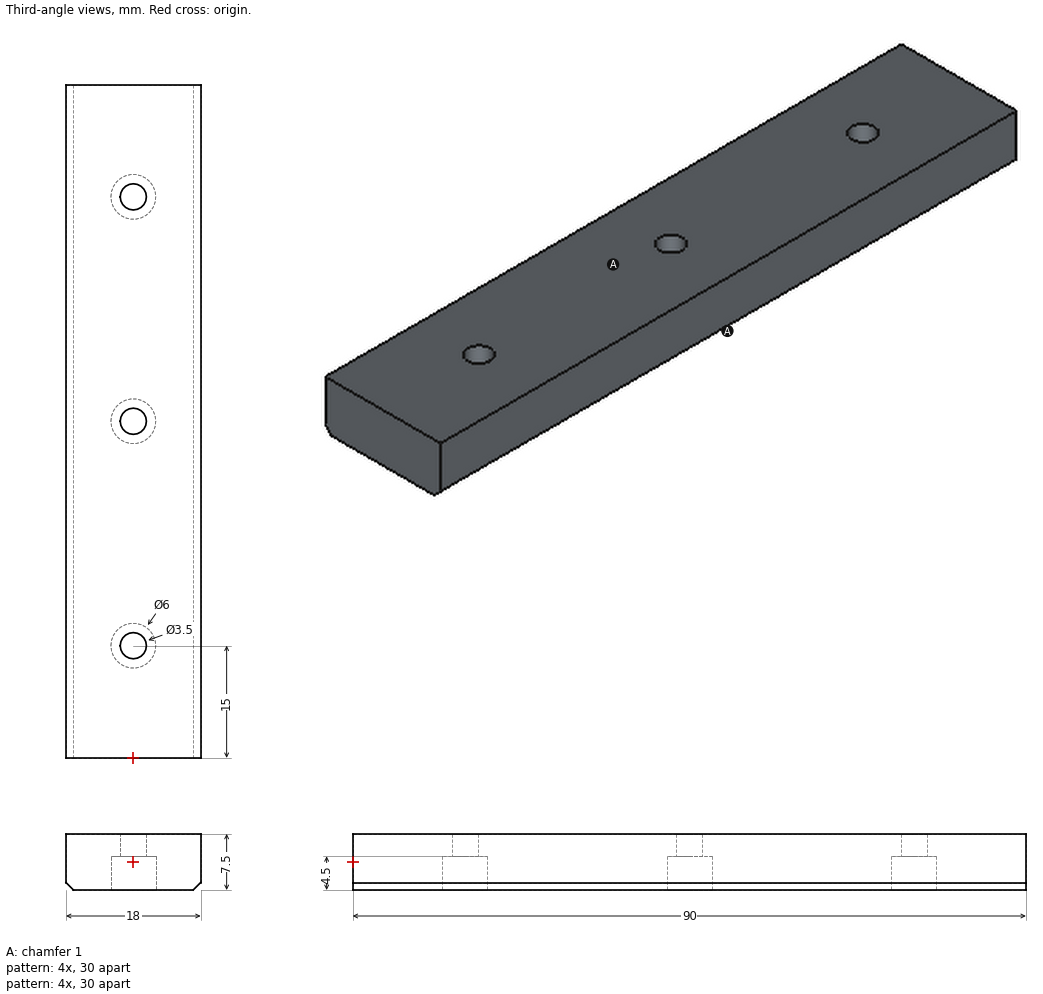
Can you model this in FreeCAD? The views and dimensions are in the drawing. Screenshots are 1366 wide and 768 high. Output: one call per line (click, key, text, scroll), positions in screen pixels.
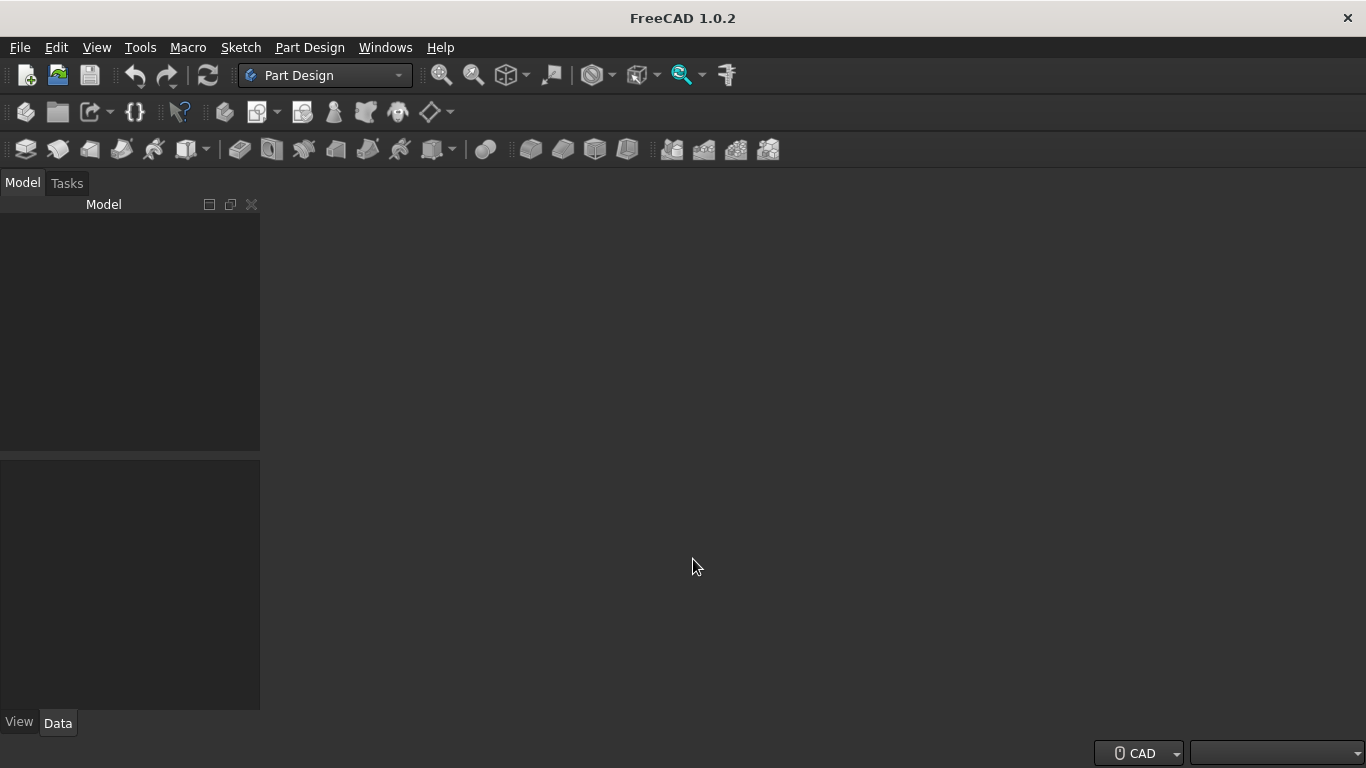
click(26, 76)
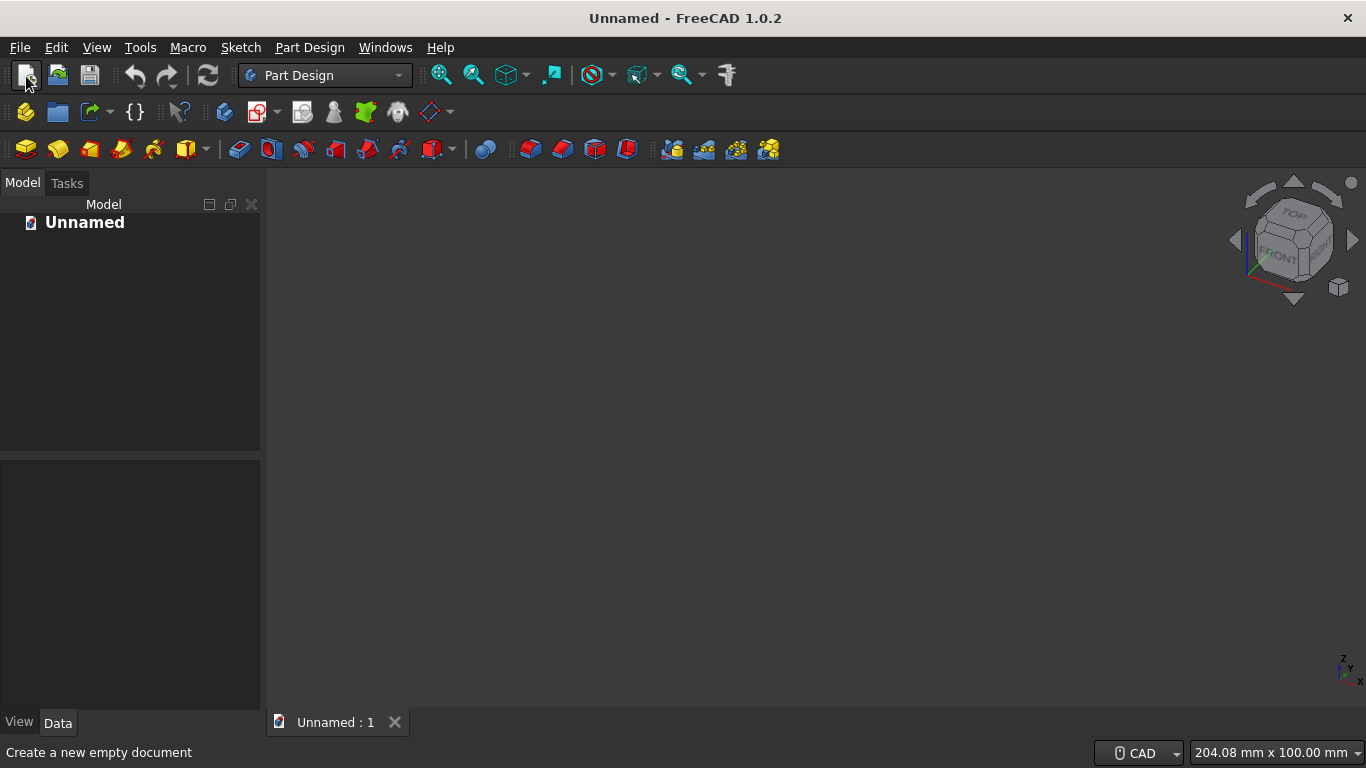
click(258, 112)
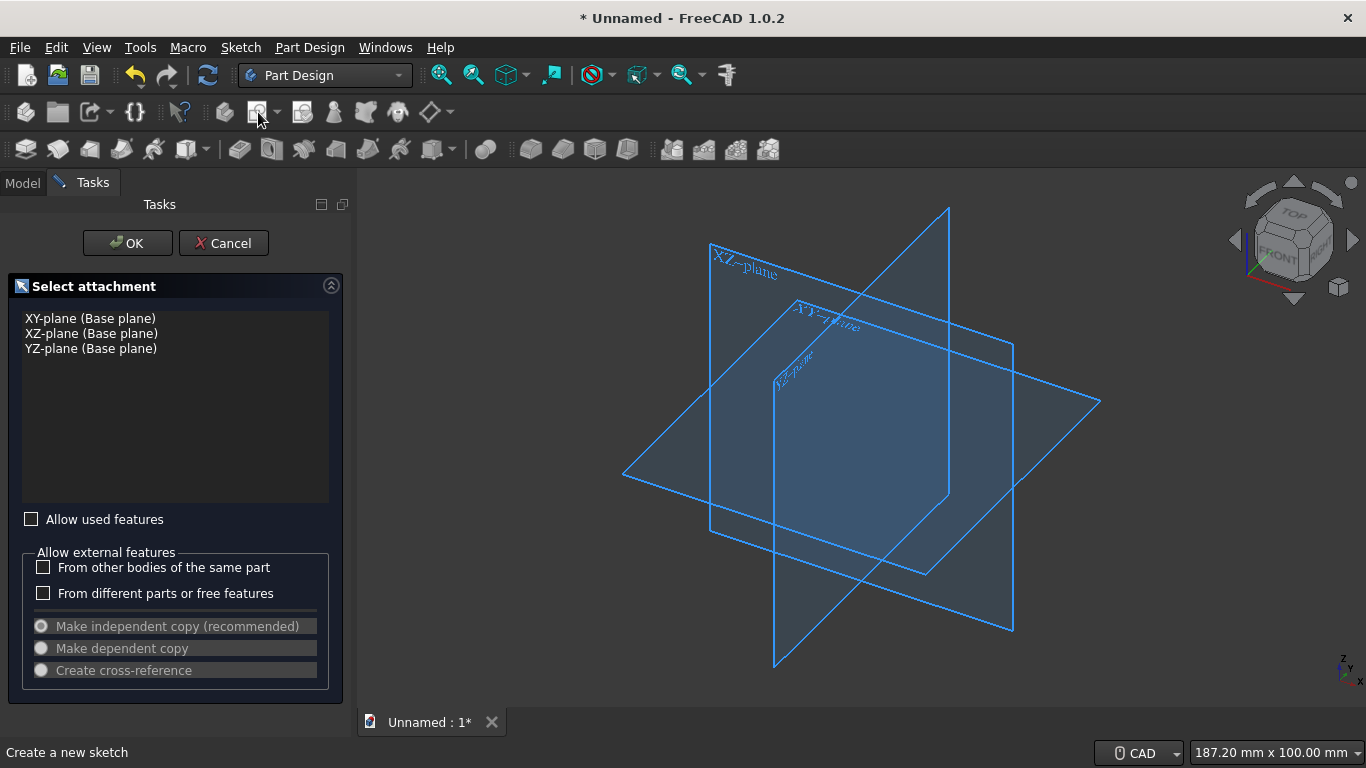
click(82, 334)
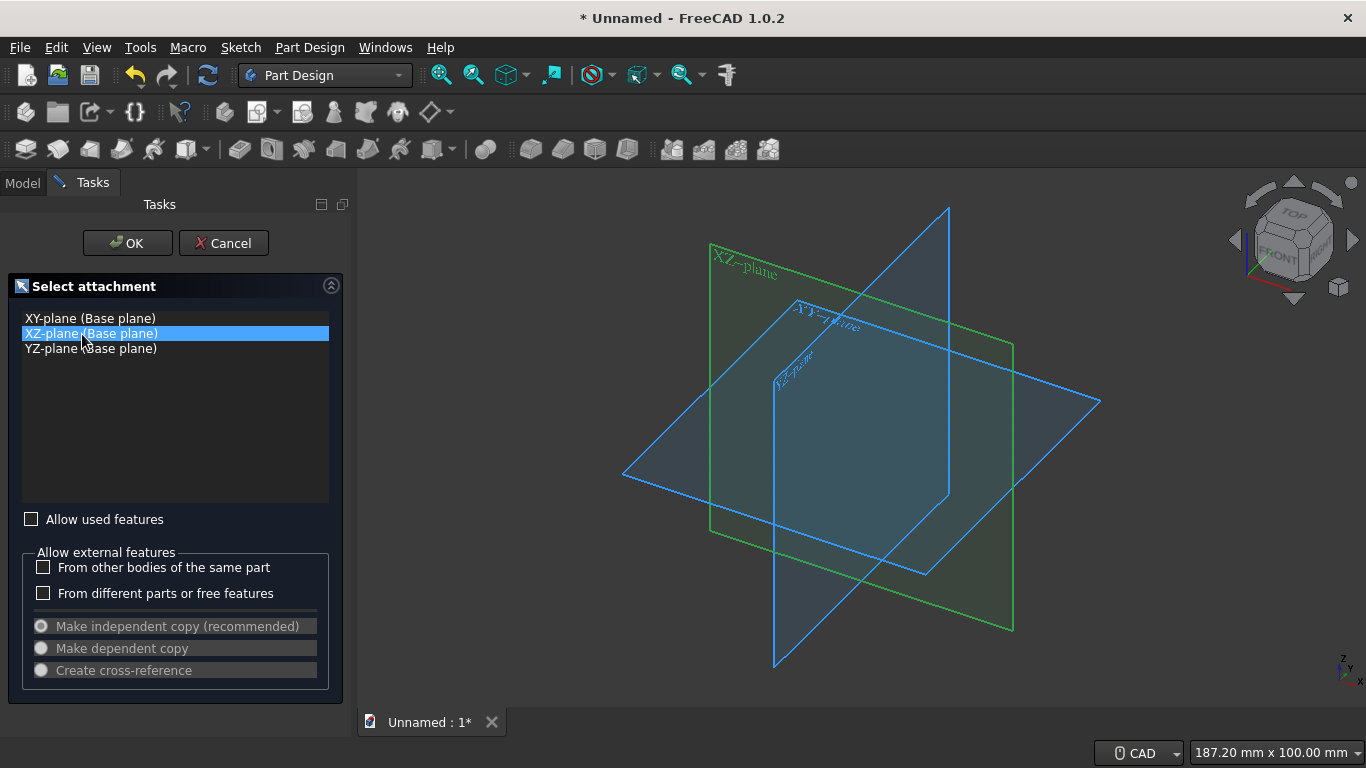
click(128, 243)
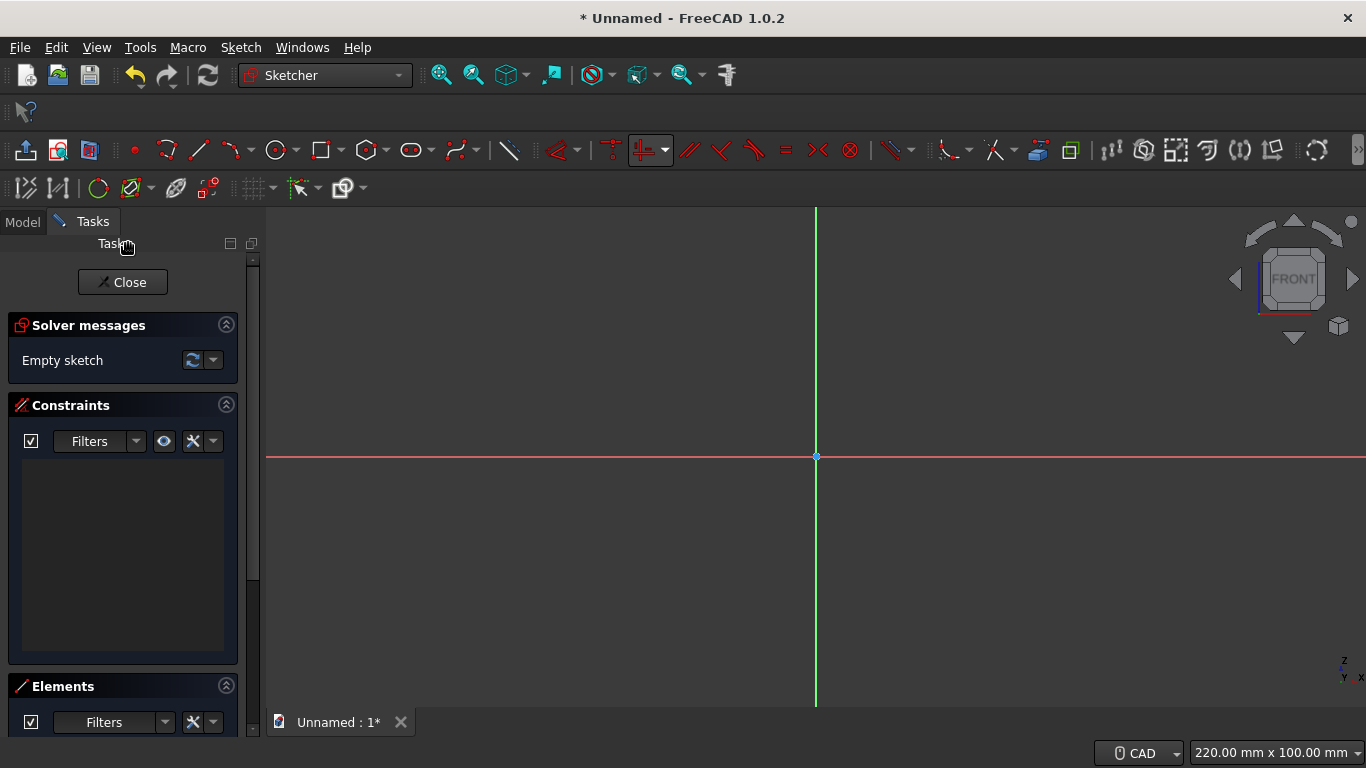
scroll(827, 457, up, 10)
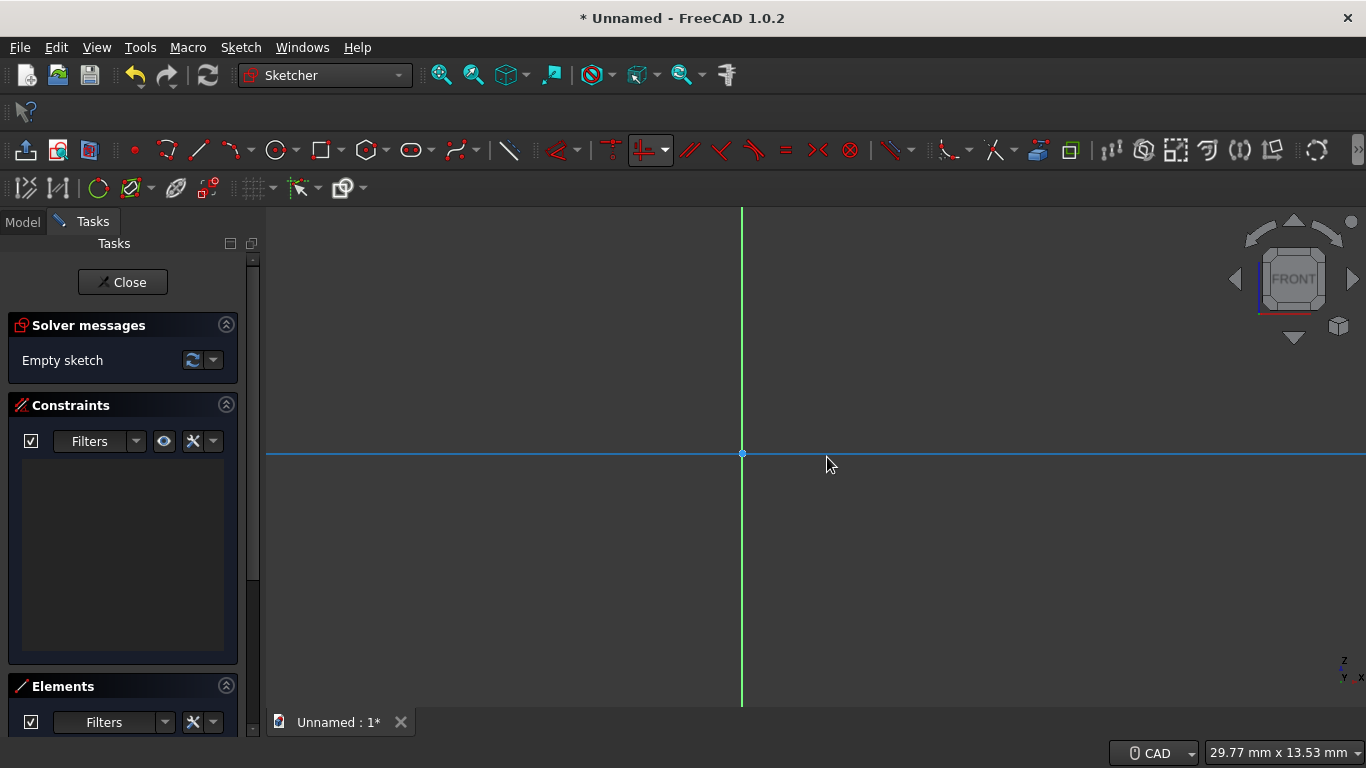
key(g)
key(v)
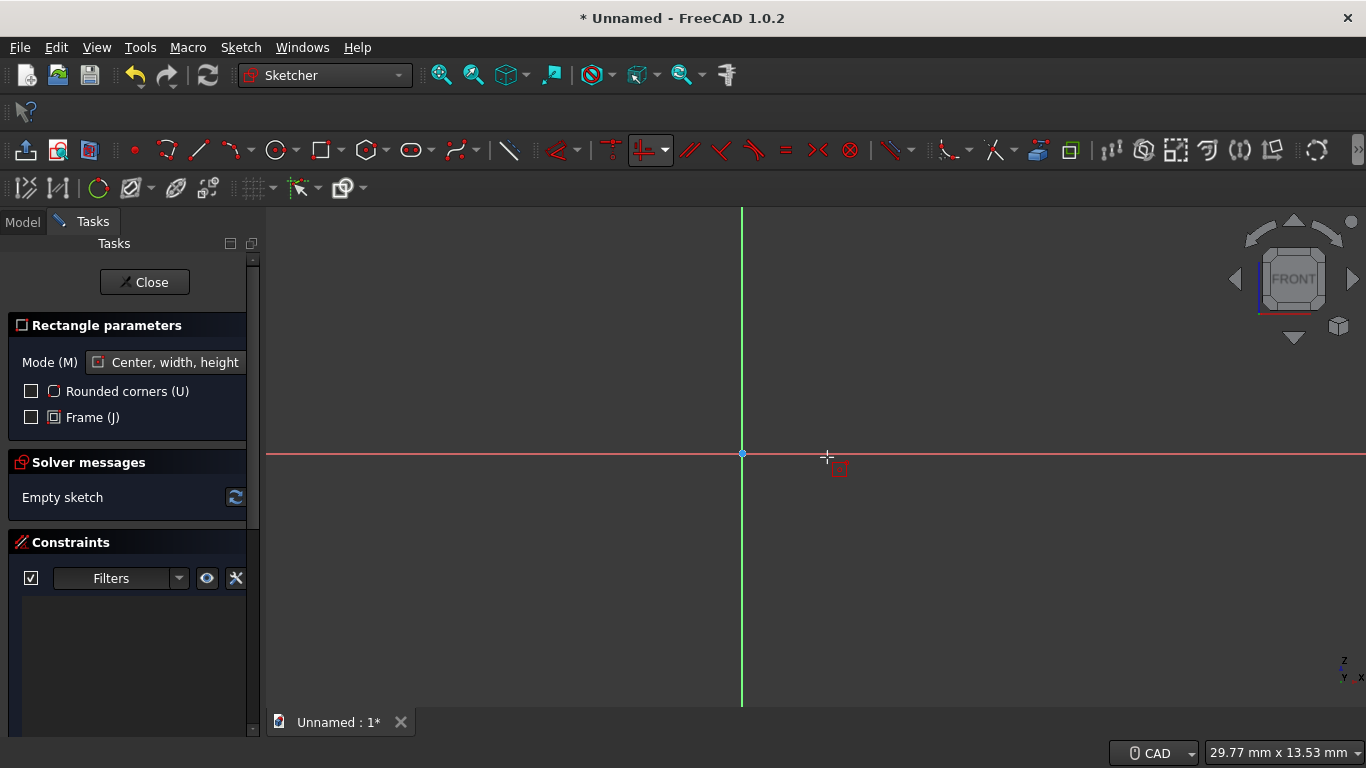
click(742, 454)
click(1075, 315)
key(Escape)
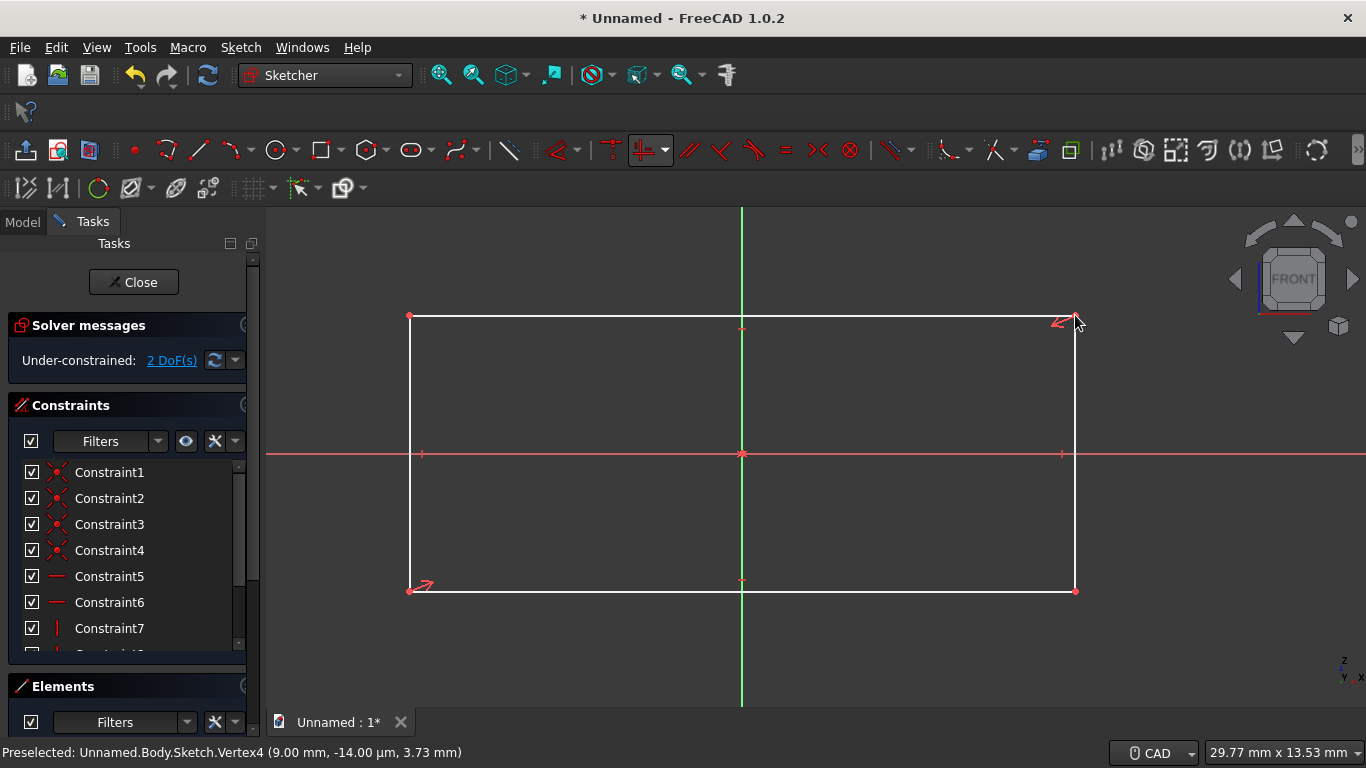
click(609, 592)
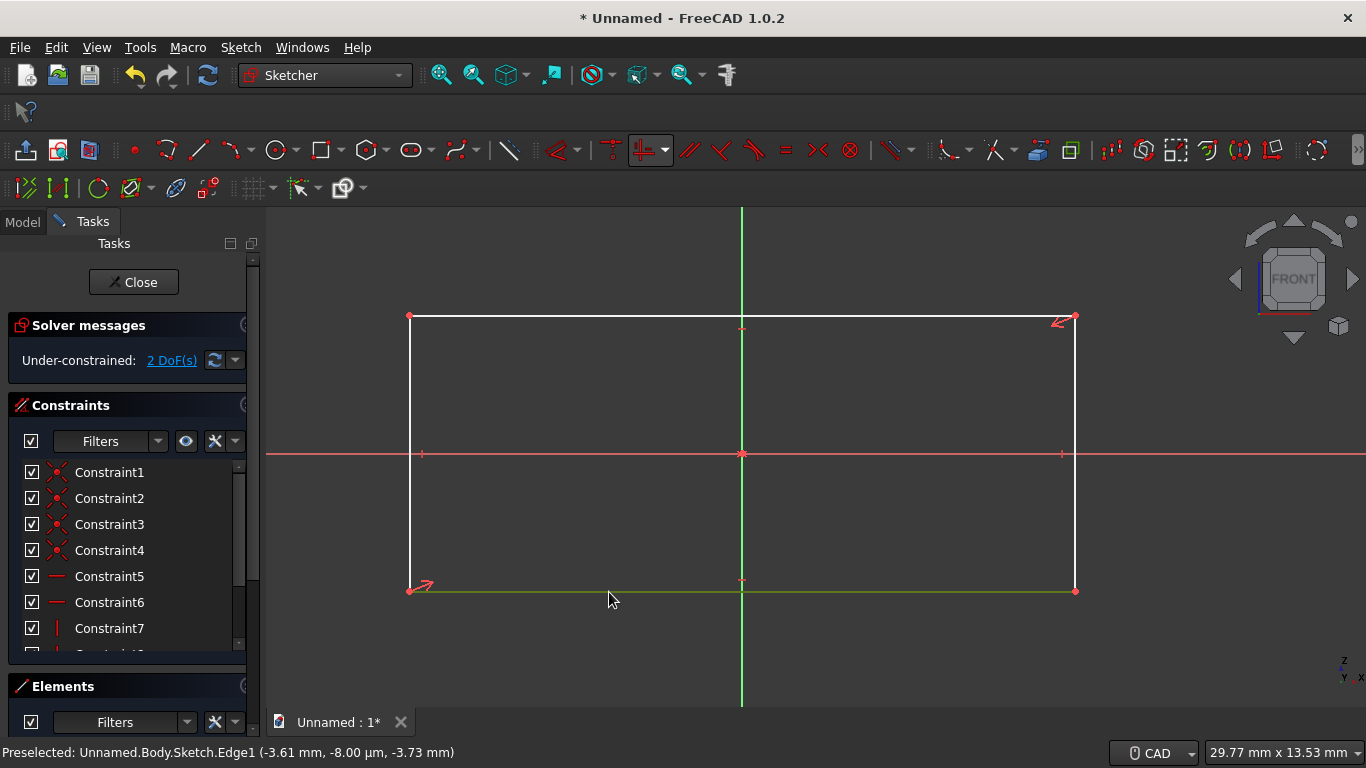
key(l)